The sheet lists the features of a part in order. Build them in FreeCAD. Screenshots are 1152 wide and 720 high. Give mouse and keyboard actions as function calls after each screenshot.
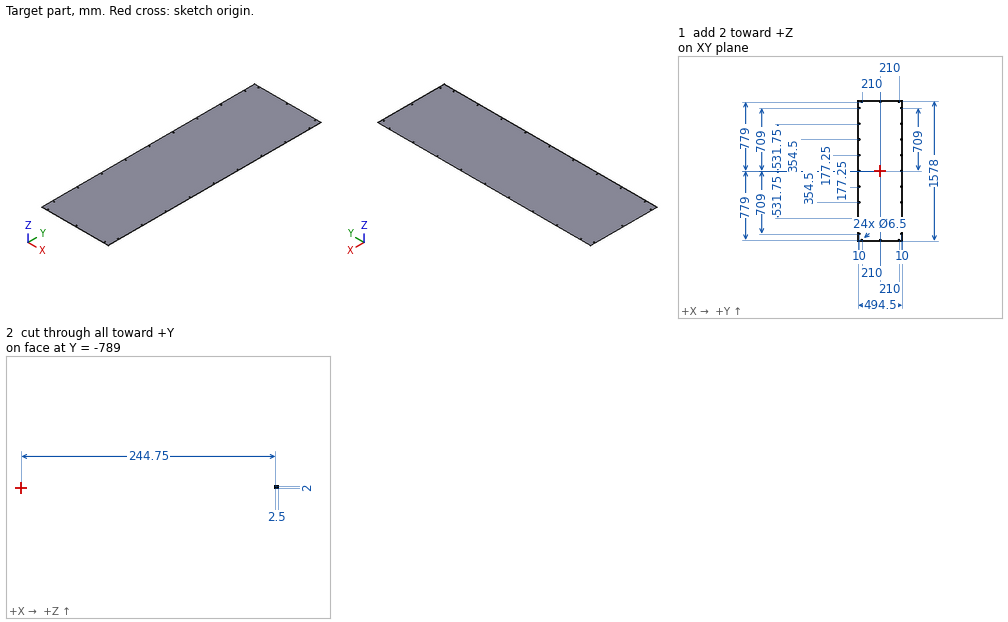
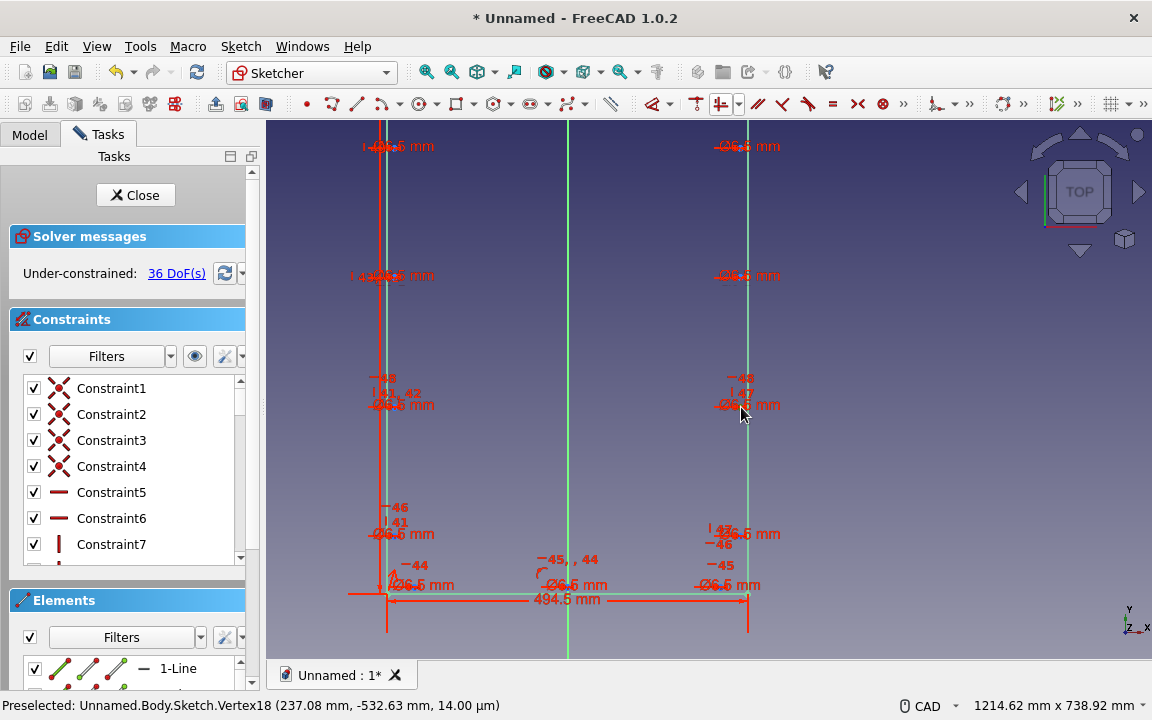
click(741, 278)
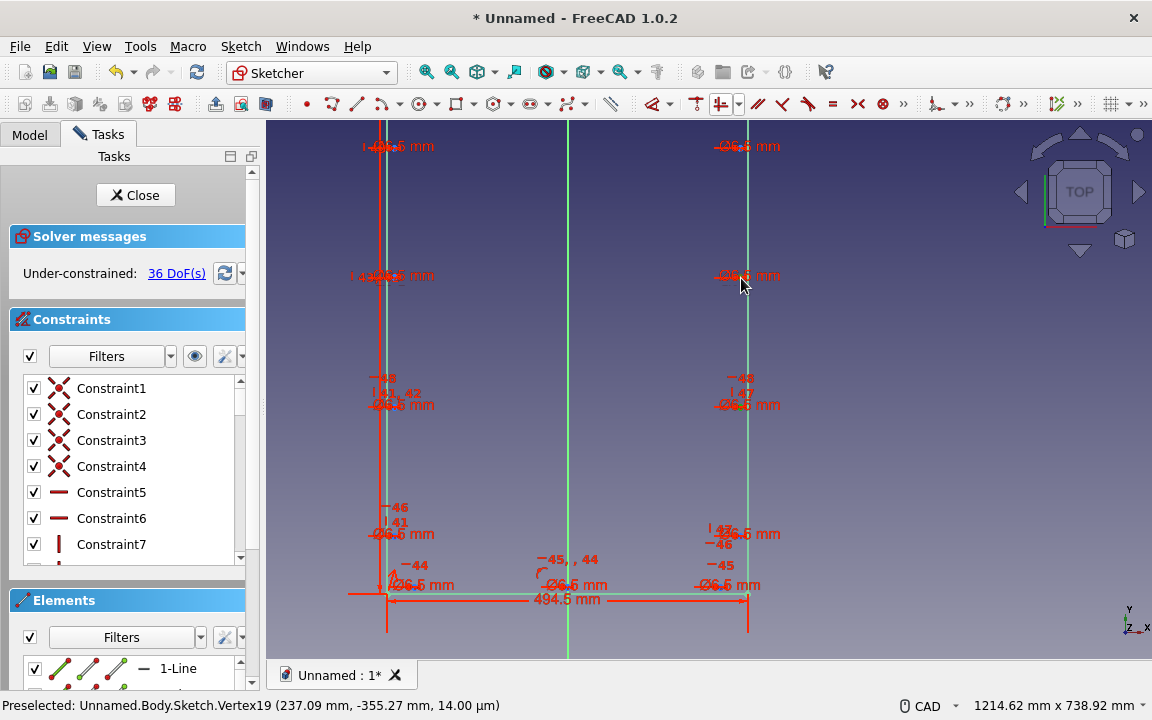
click(738, 104)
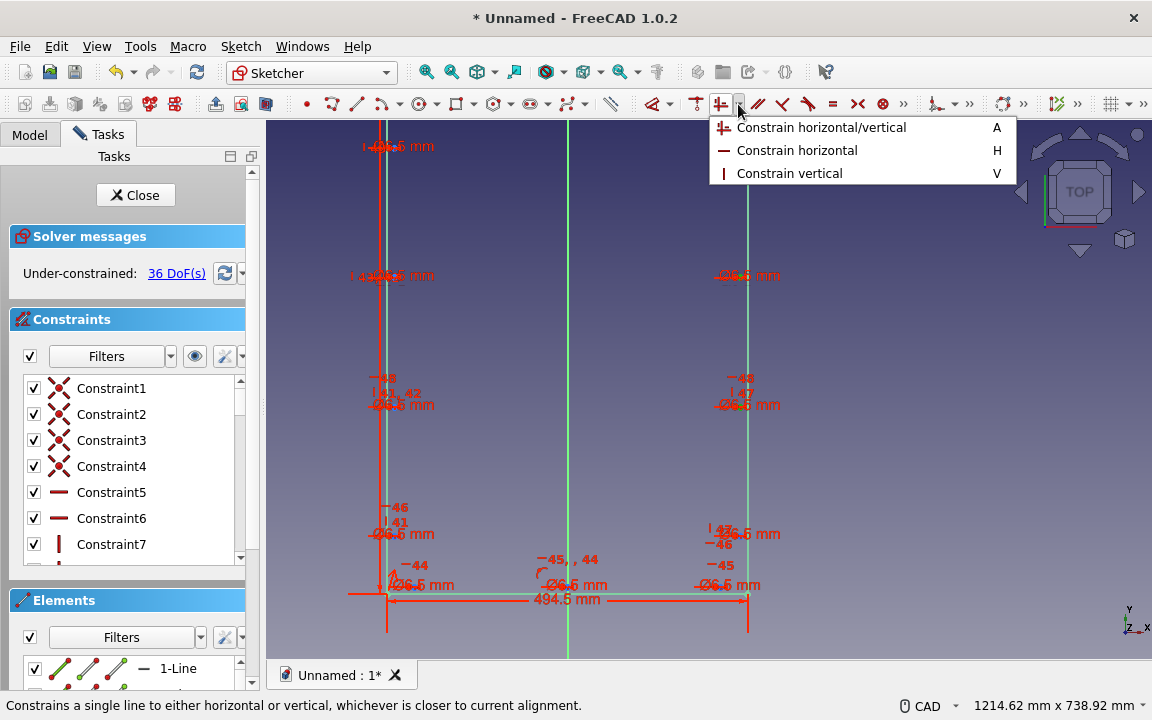
click(863, 174)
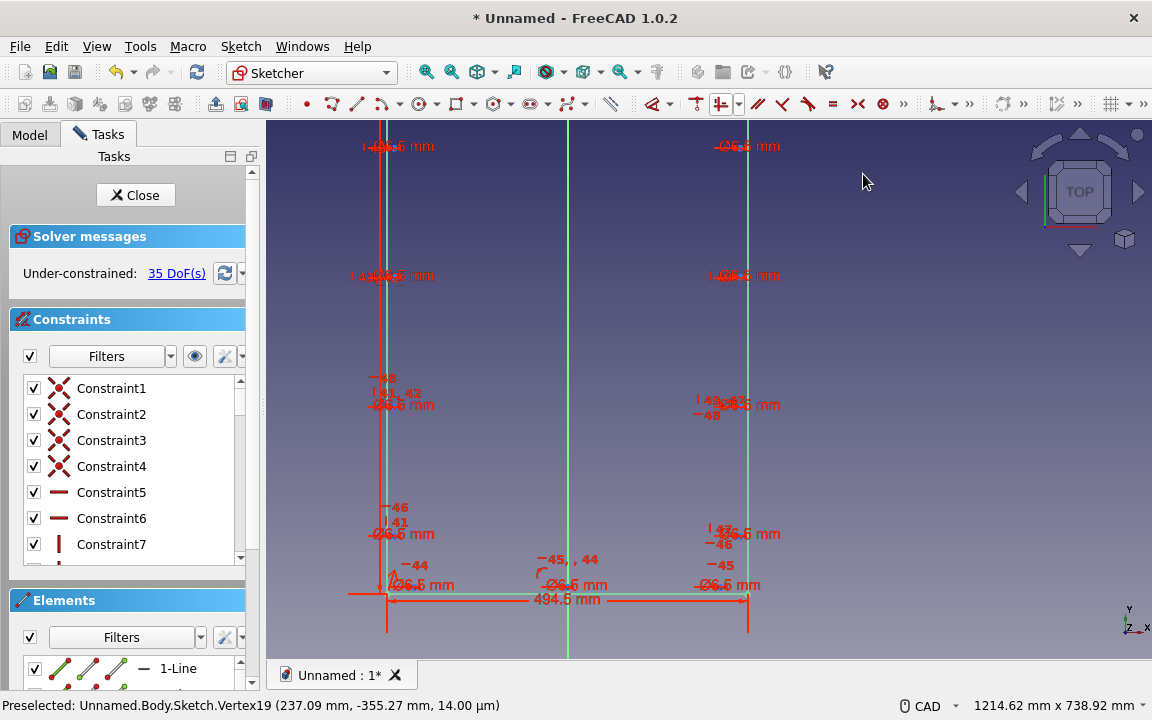
click(394, 278)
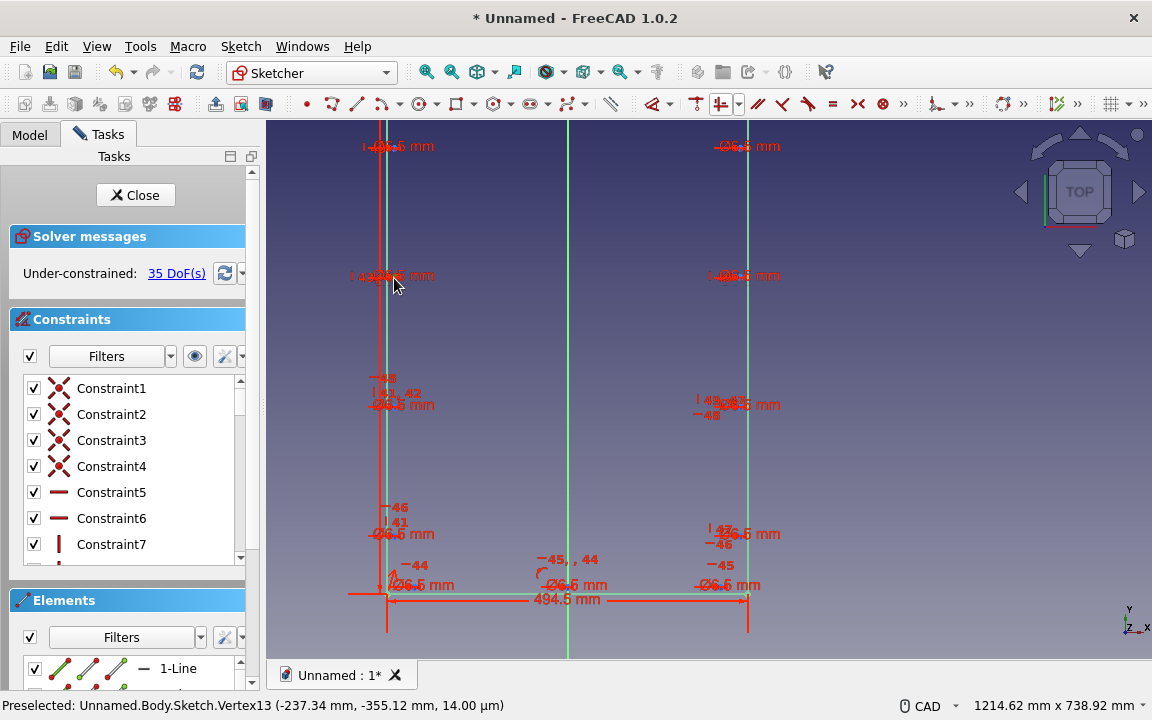
click(741, 278)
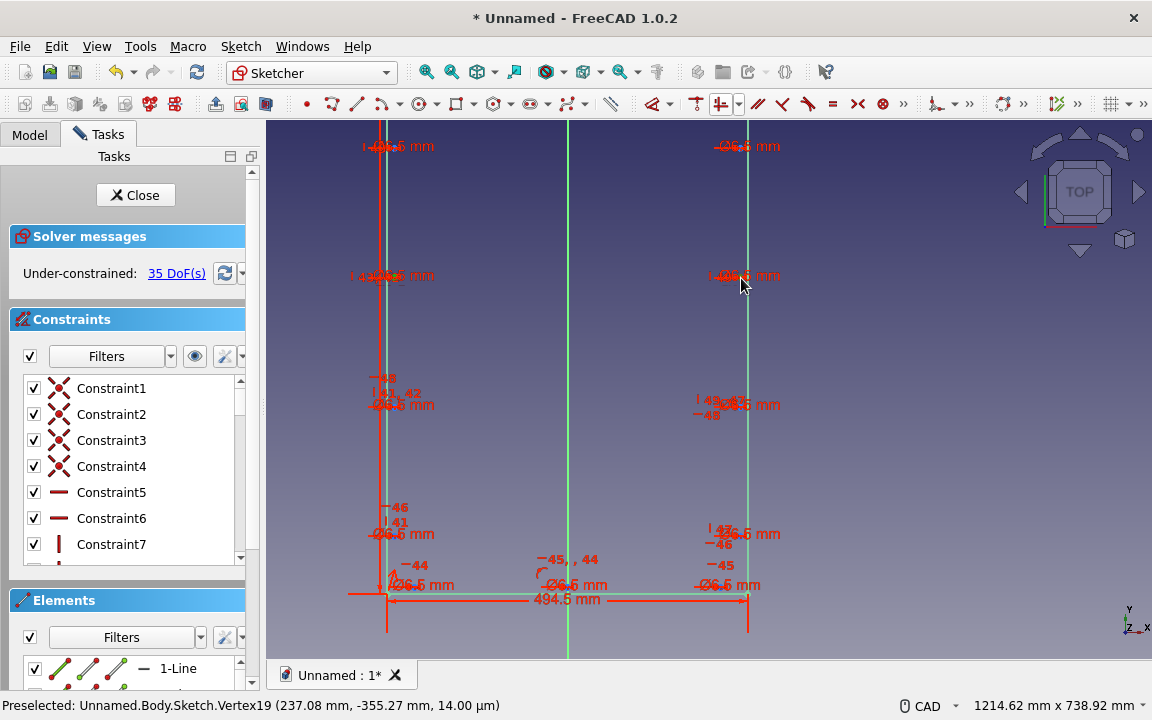
click(738, 104)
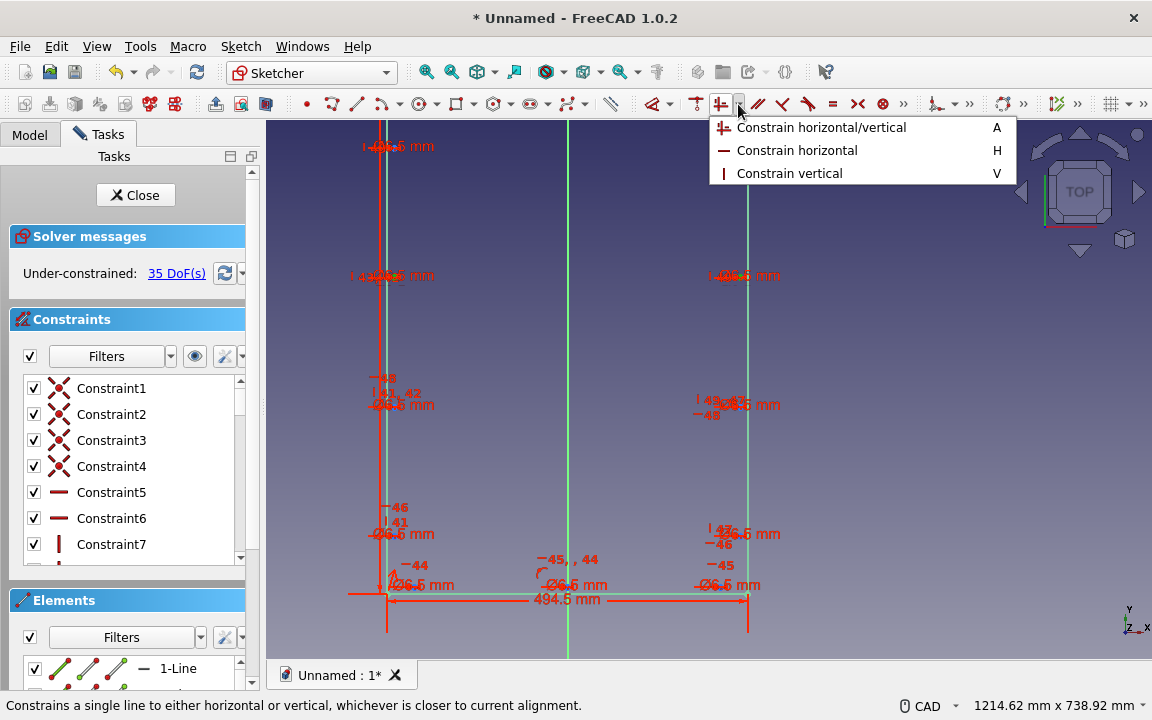
click(863, 150)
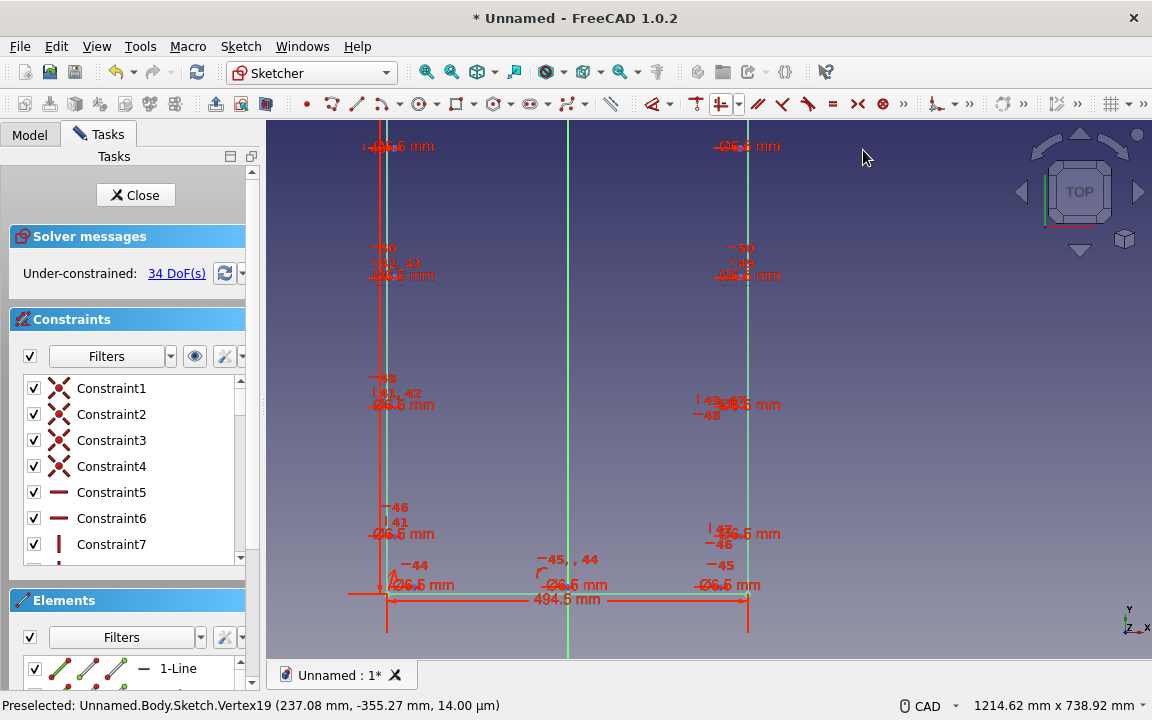
click(741, 278)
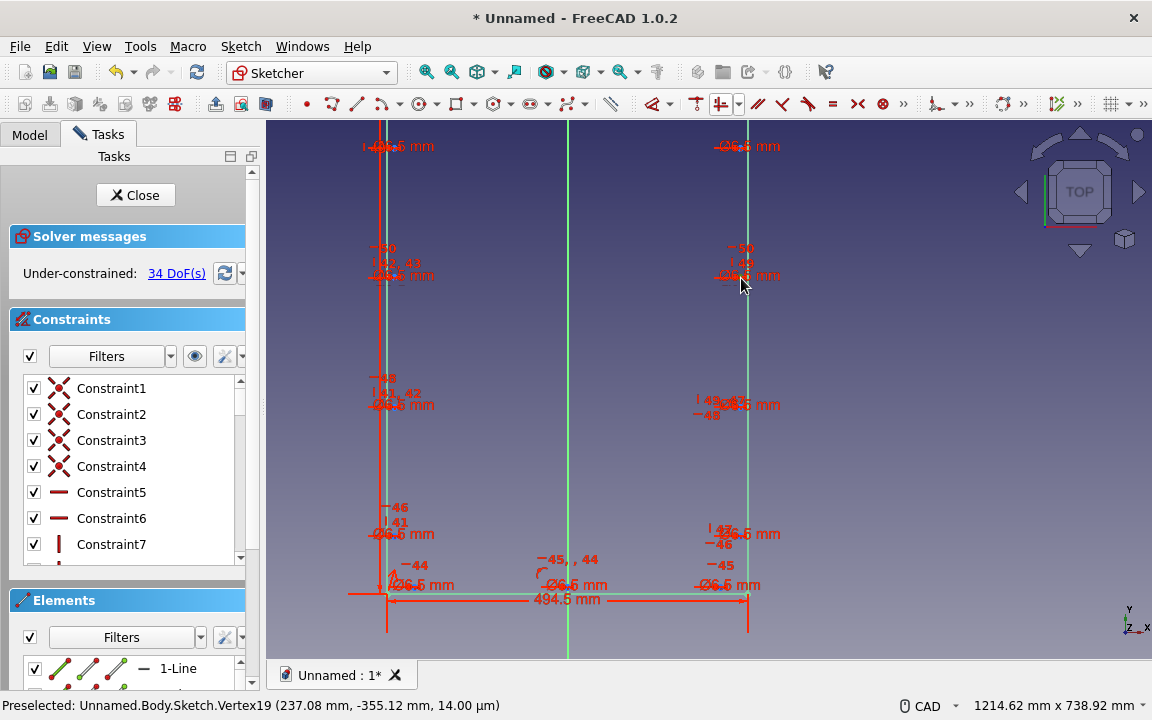
click(741, 148)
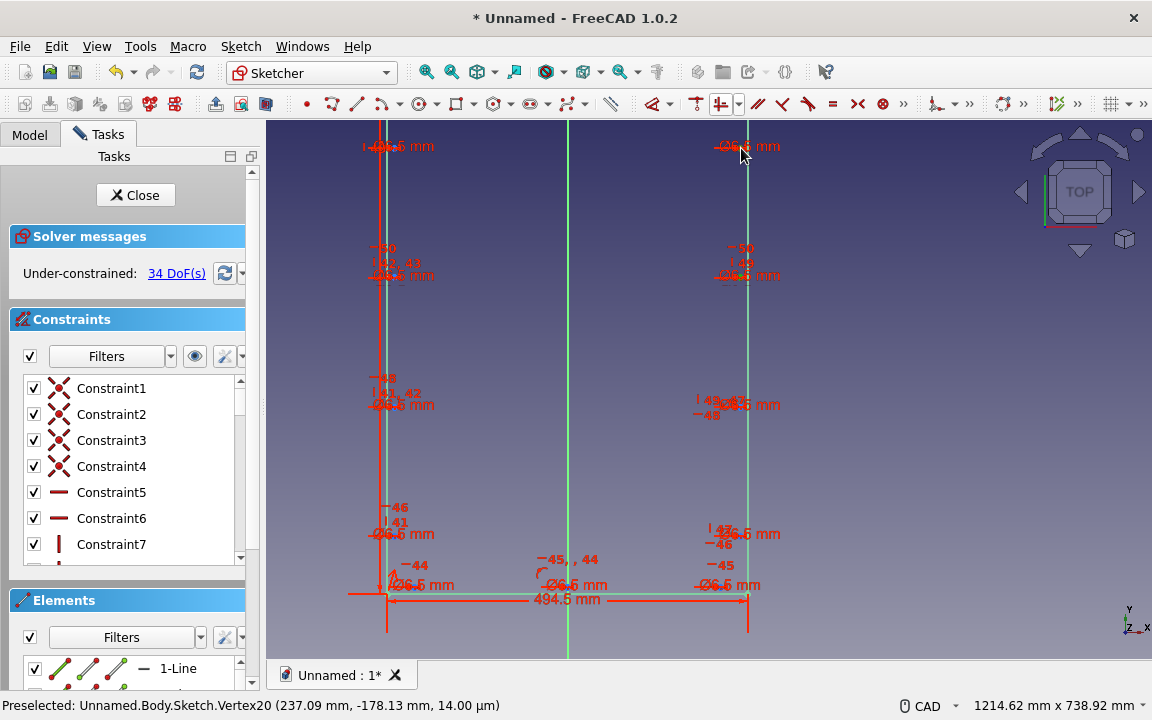
click(738, 104)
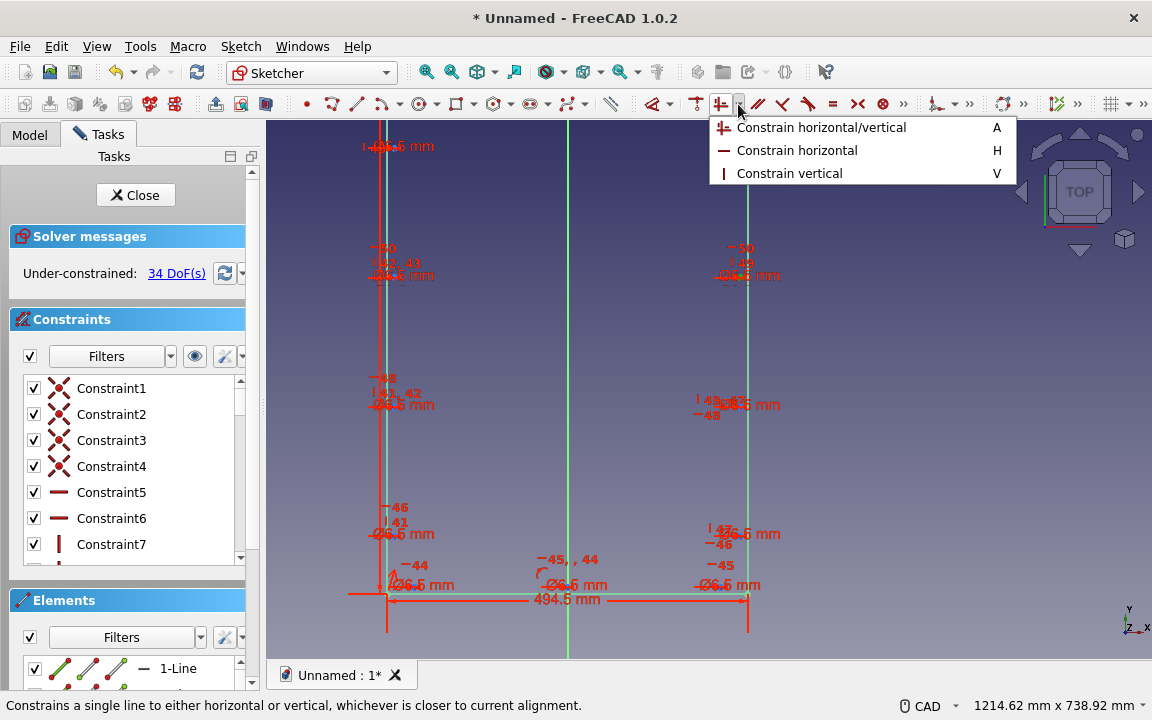
click(863, 174)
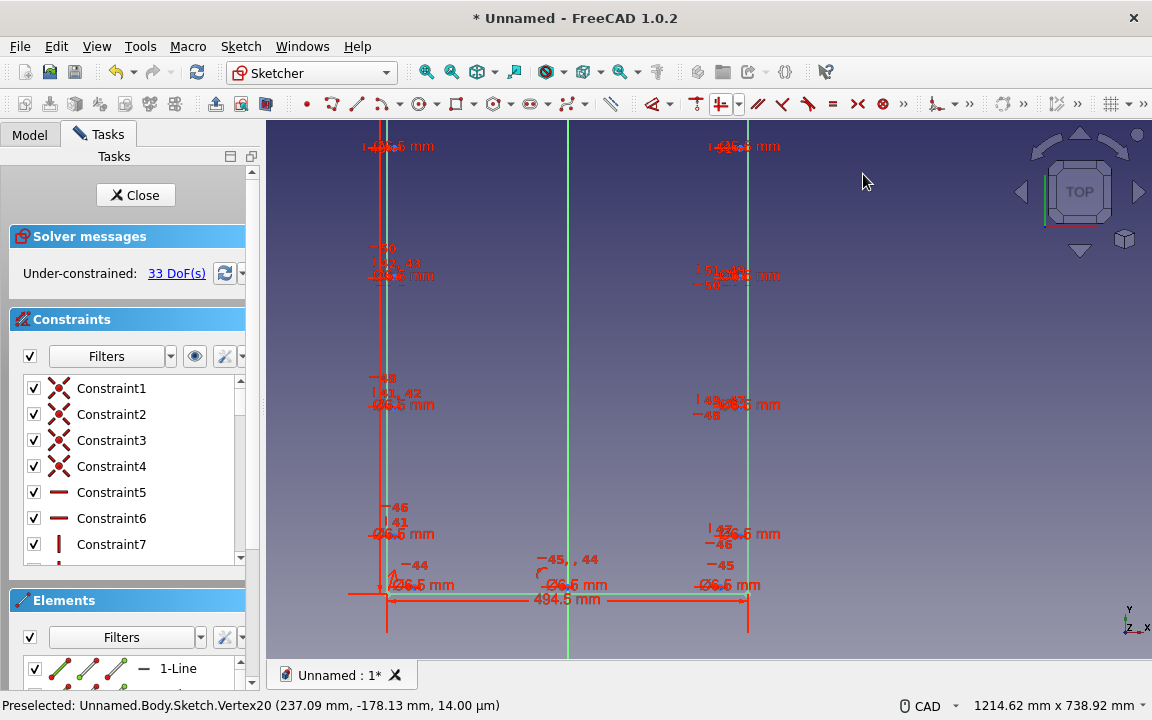
click(394, 148)